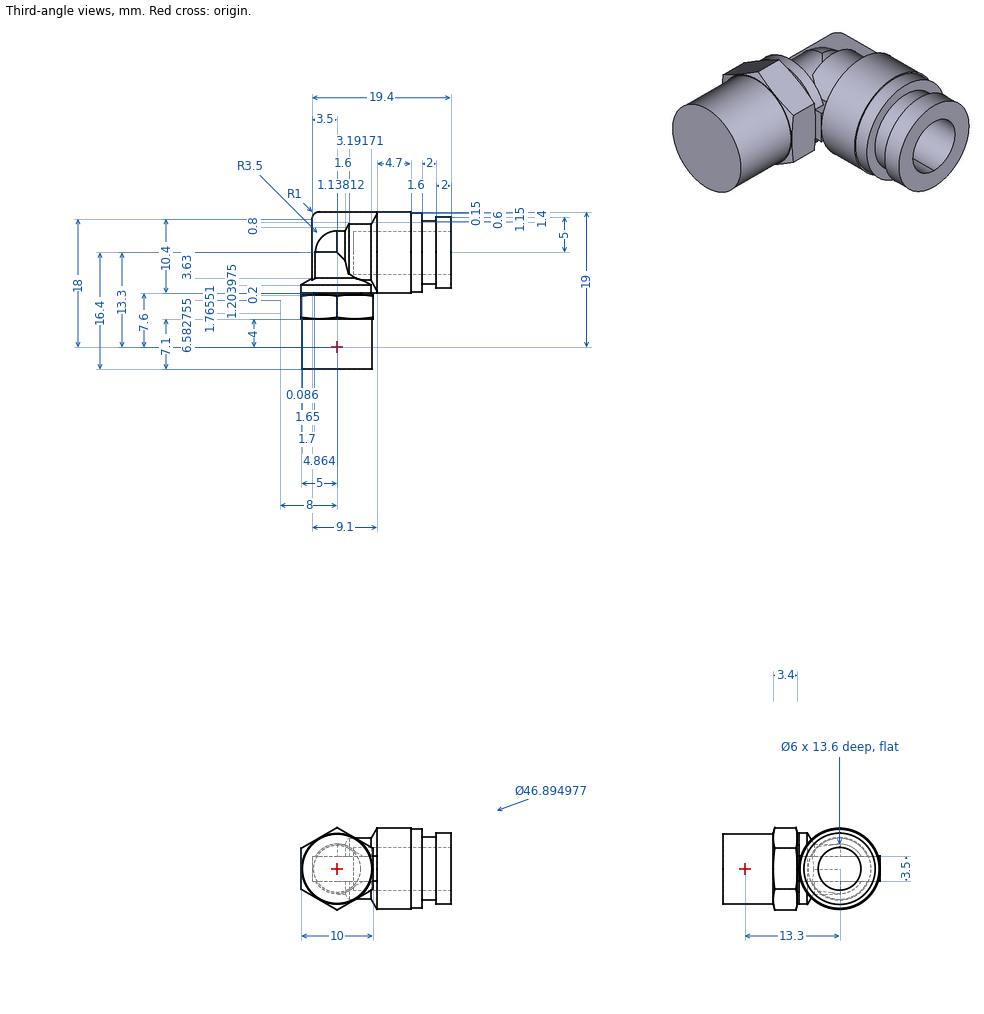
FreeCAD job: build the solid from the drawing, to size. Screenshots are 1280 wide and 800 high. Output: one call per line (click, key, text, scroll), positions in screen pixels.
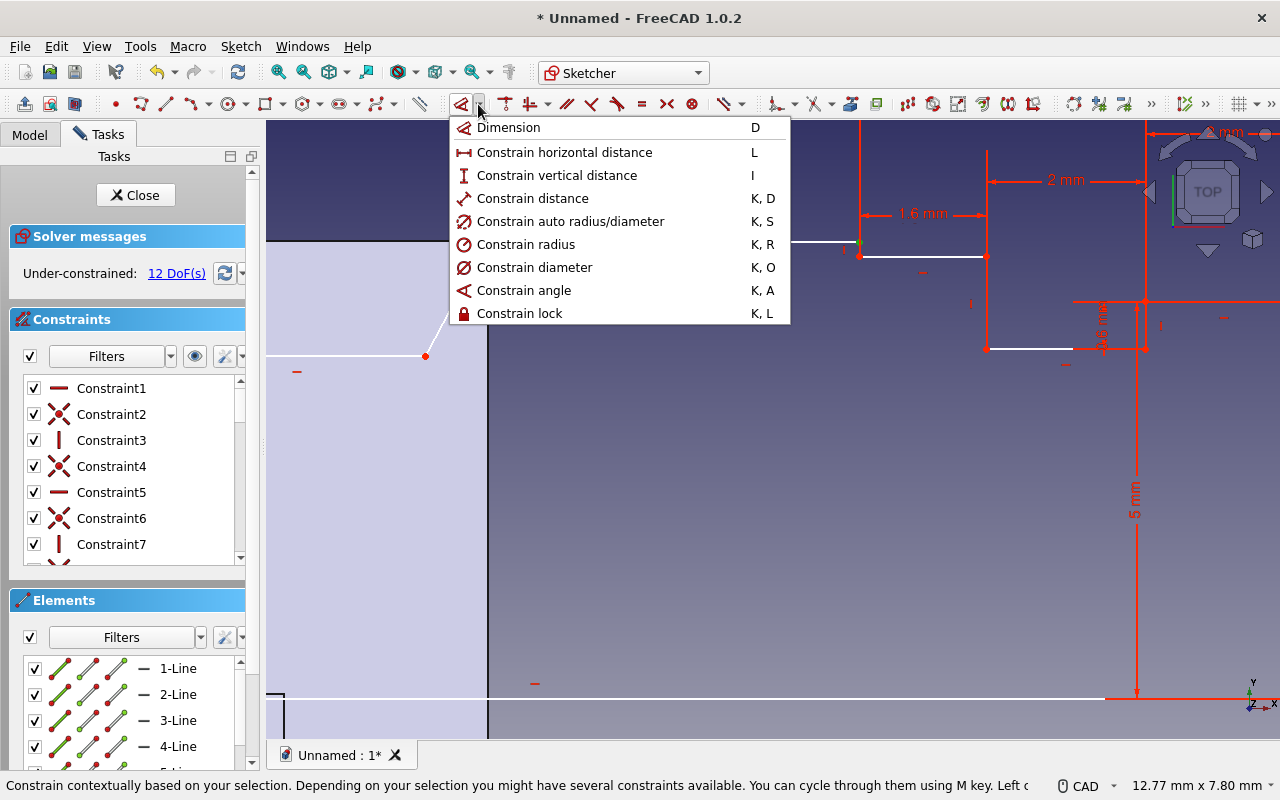
click(620, 176)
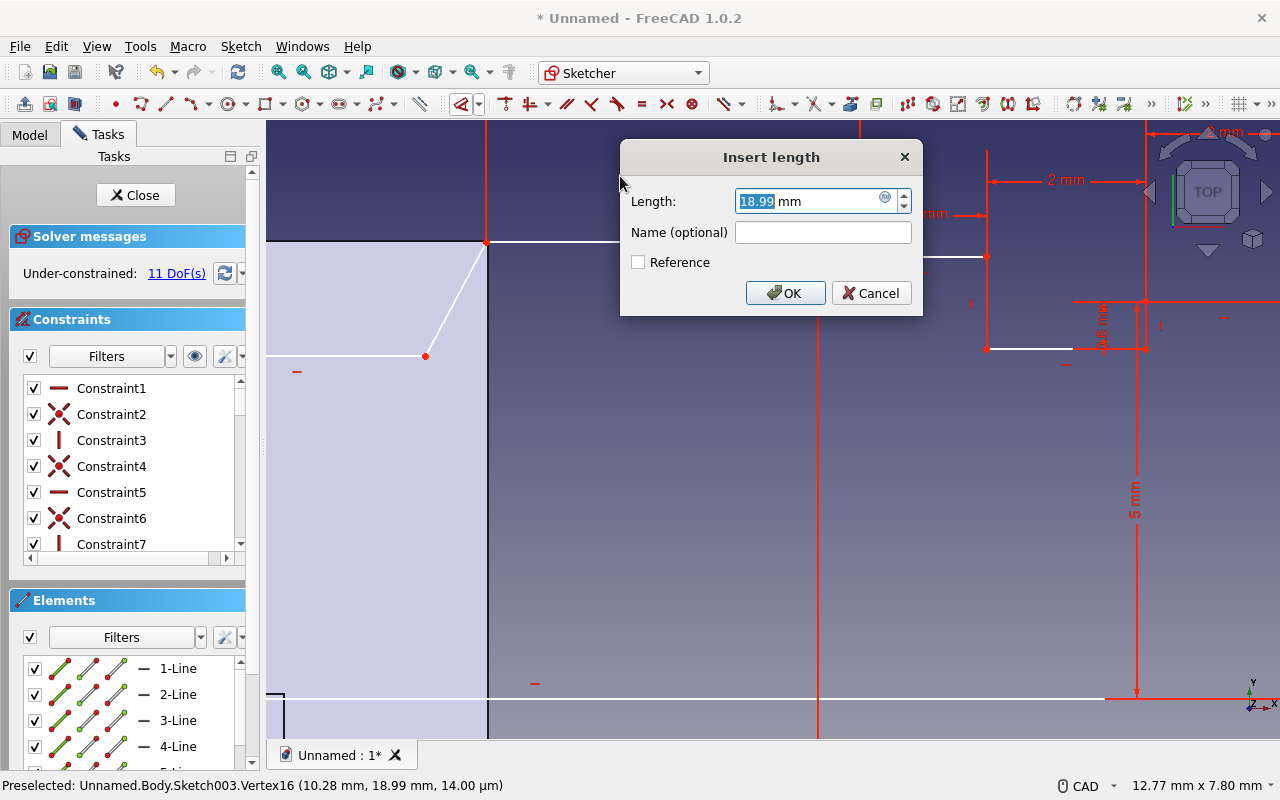
text(19)
key(Return)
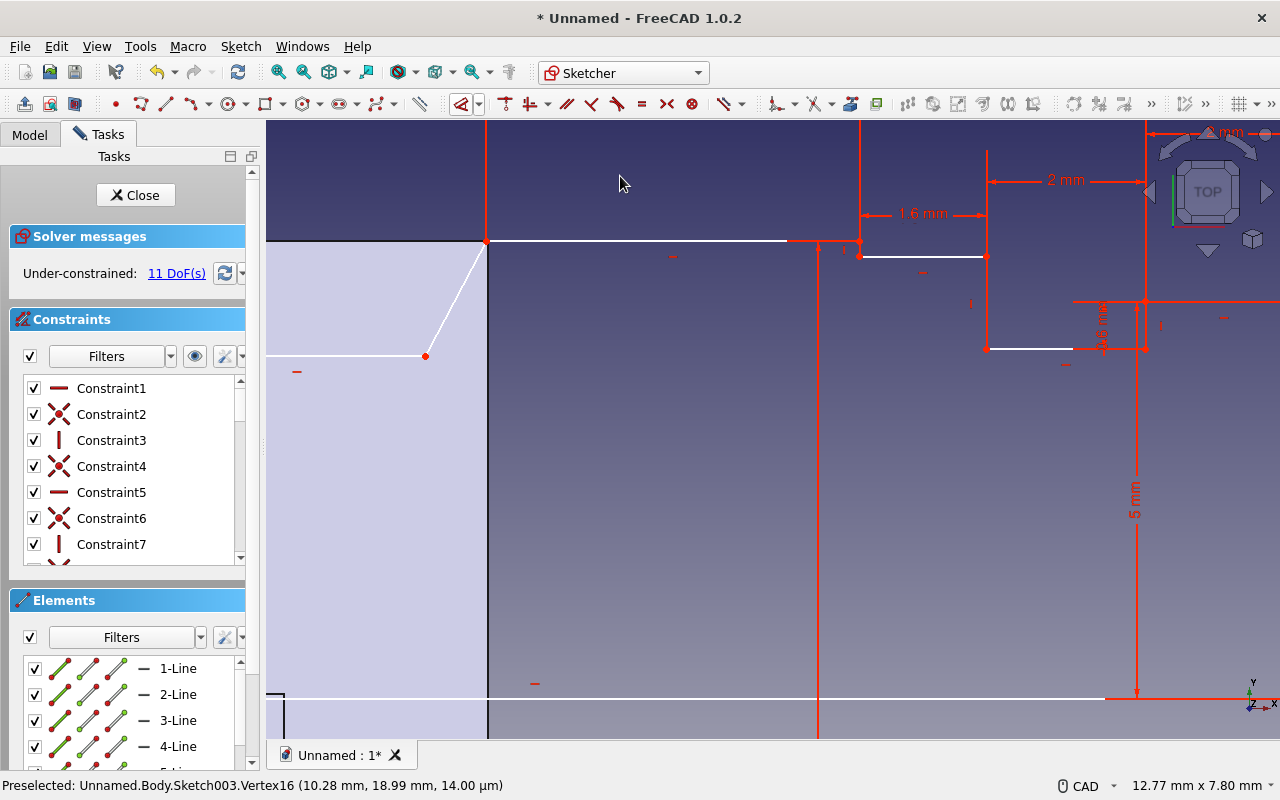
scroll(861, 244, down, 7)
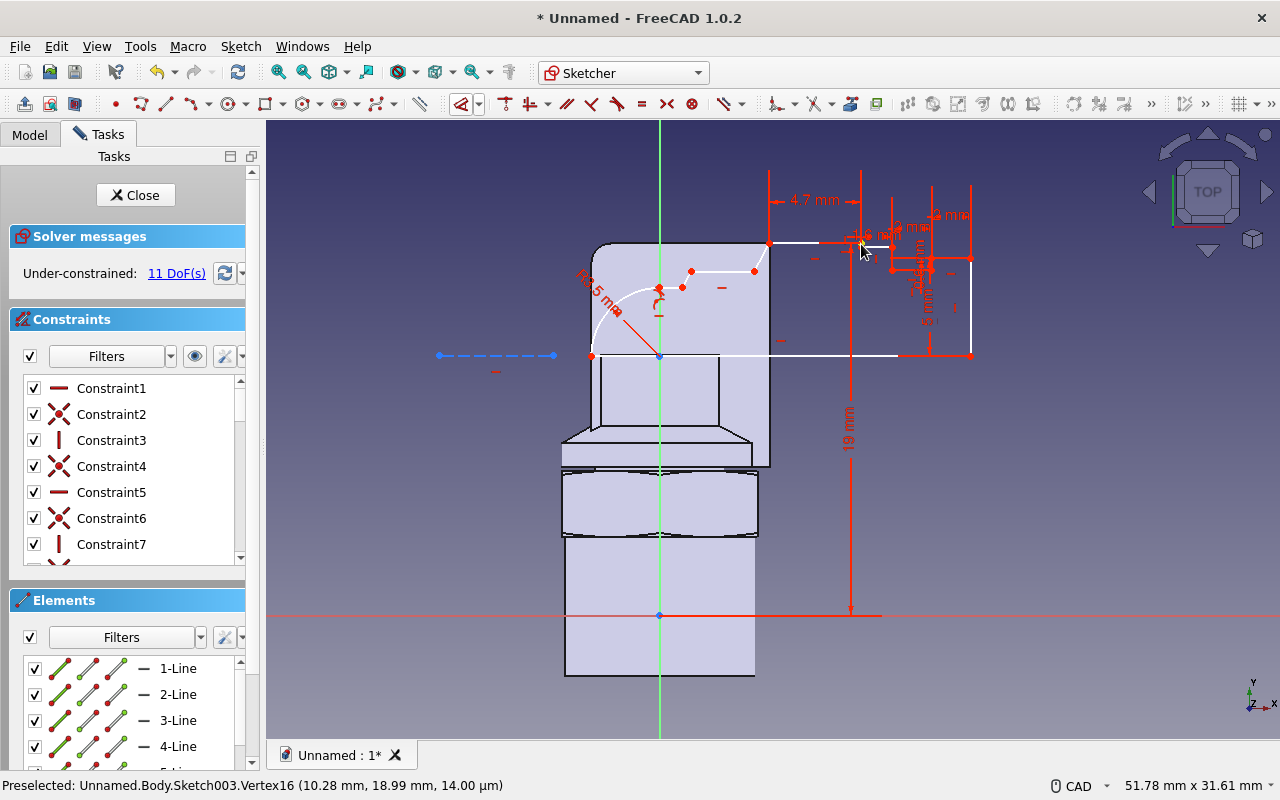
click(857, 356)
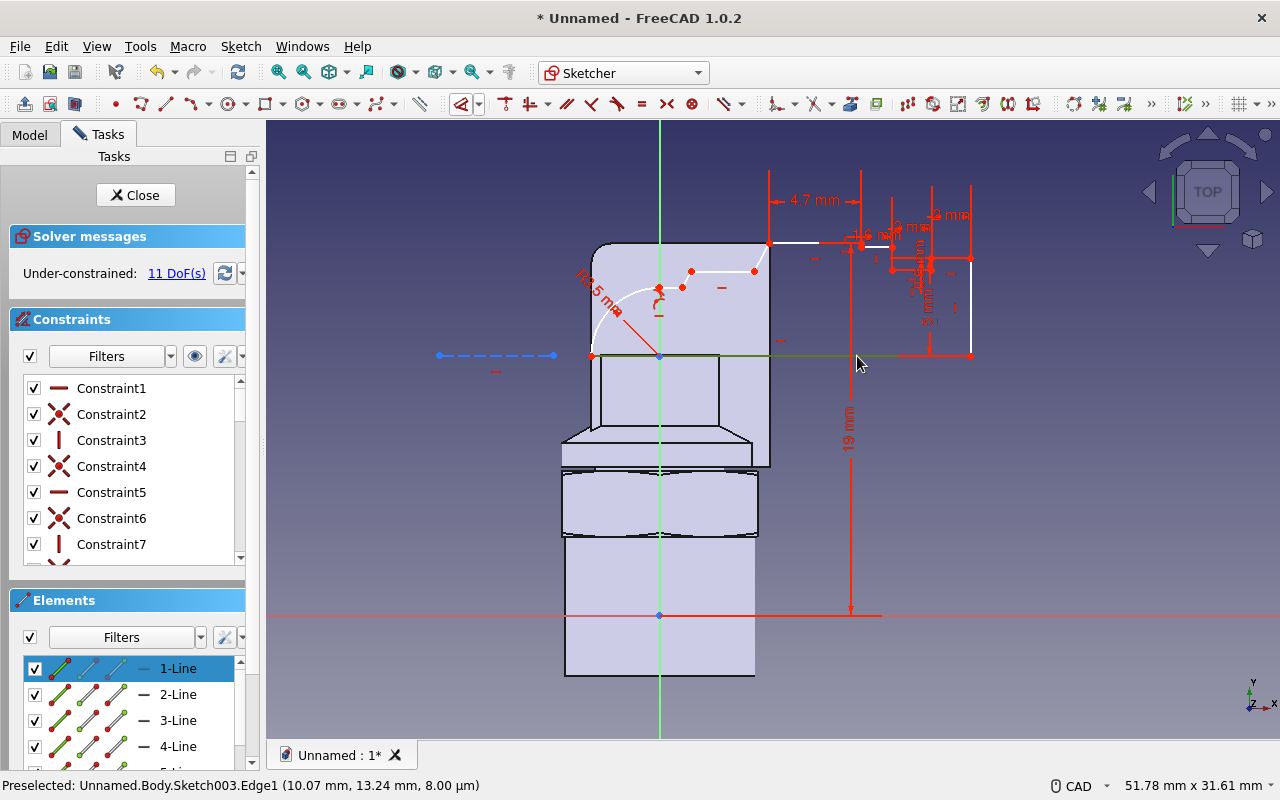
key(l)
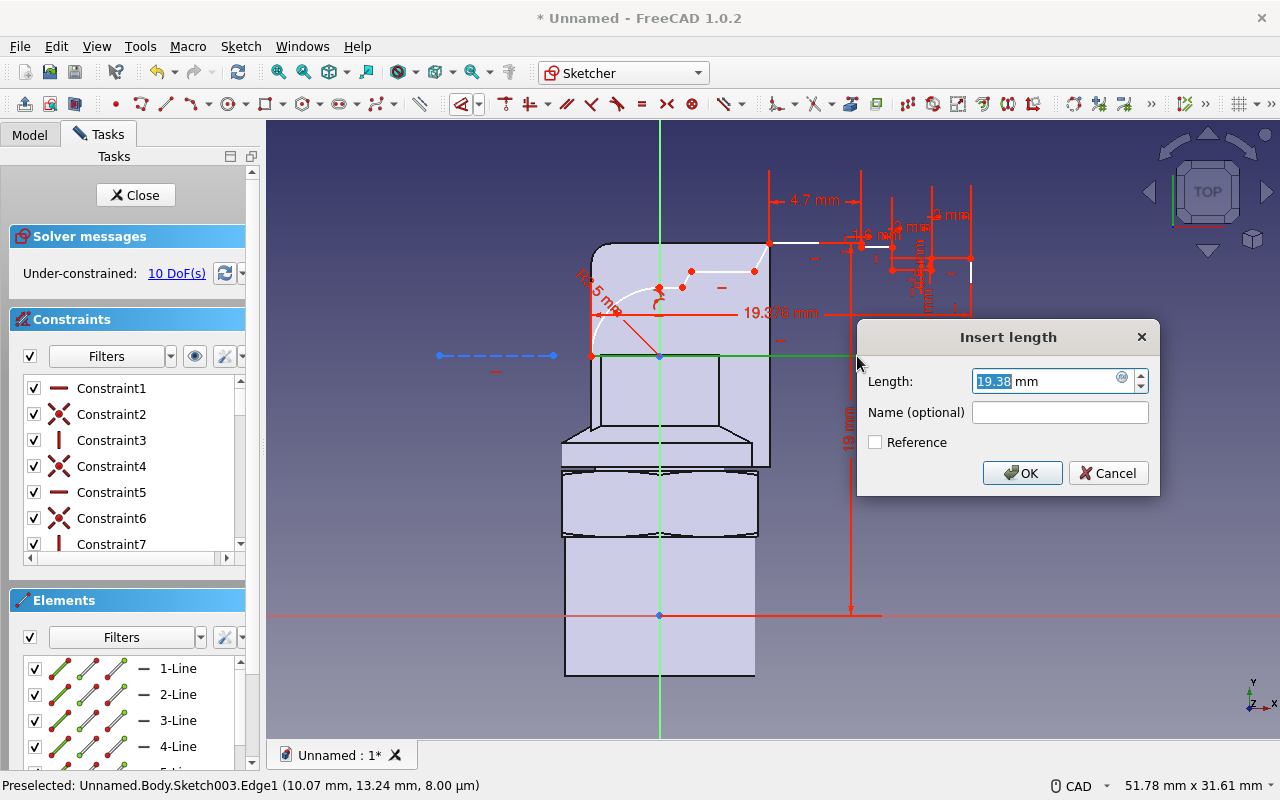
text(19.4)
key(Return)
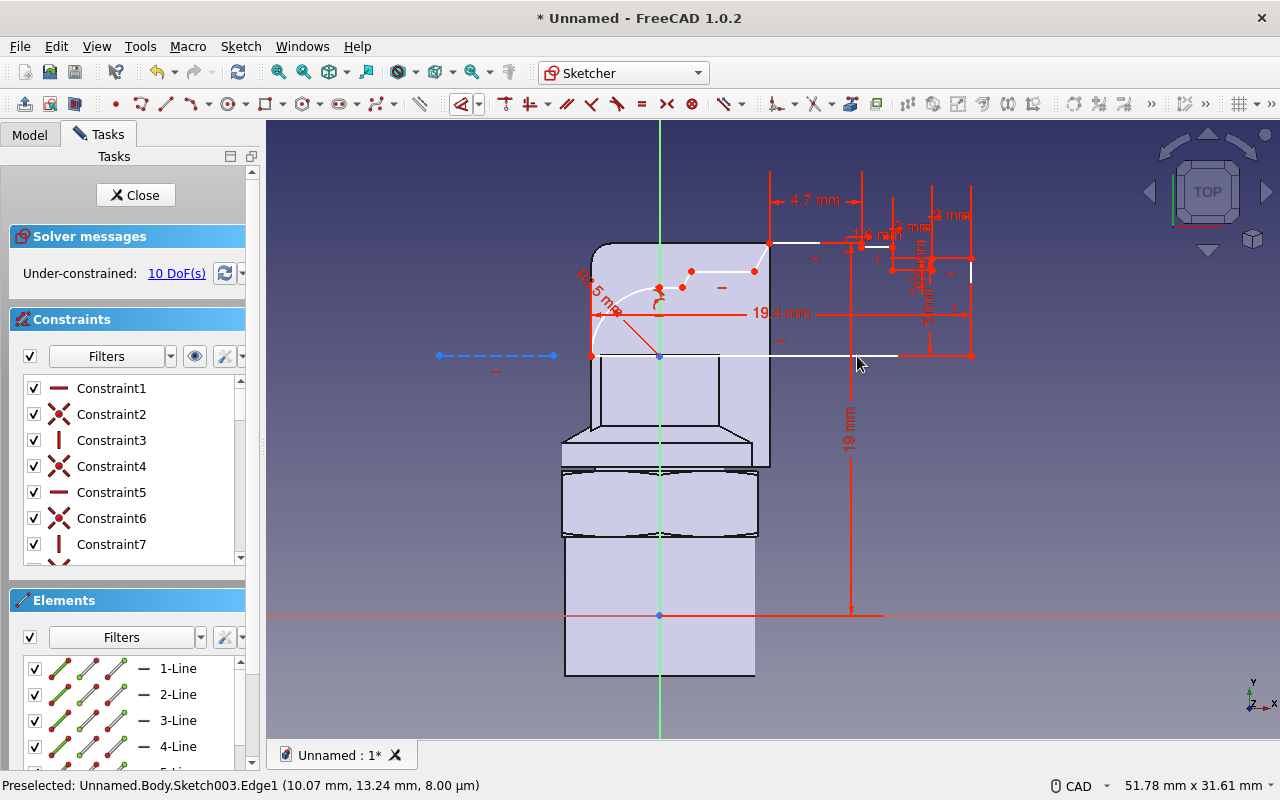
scroll(893, 261, up, 3)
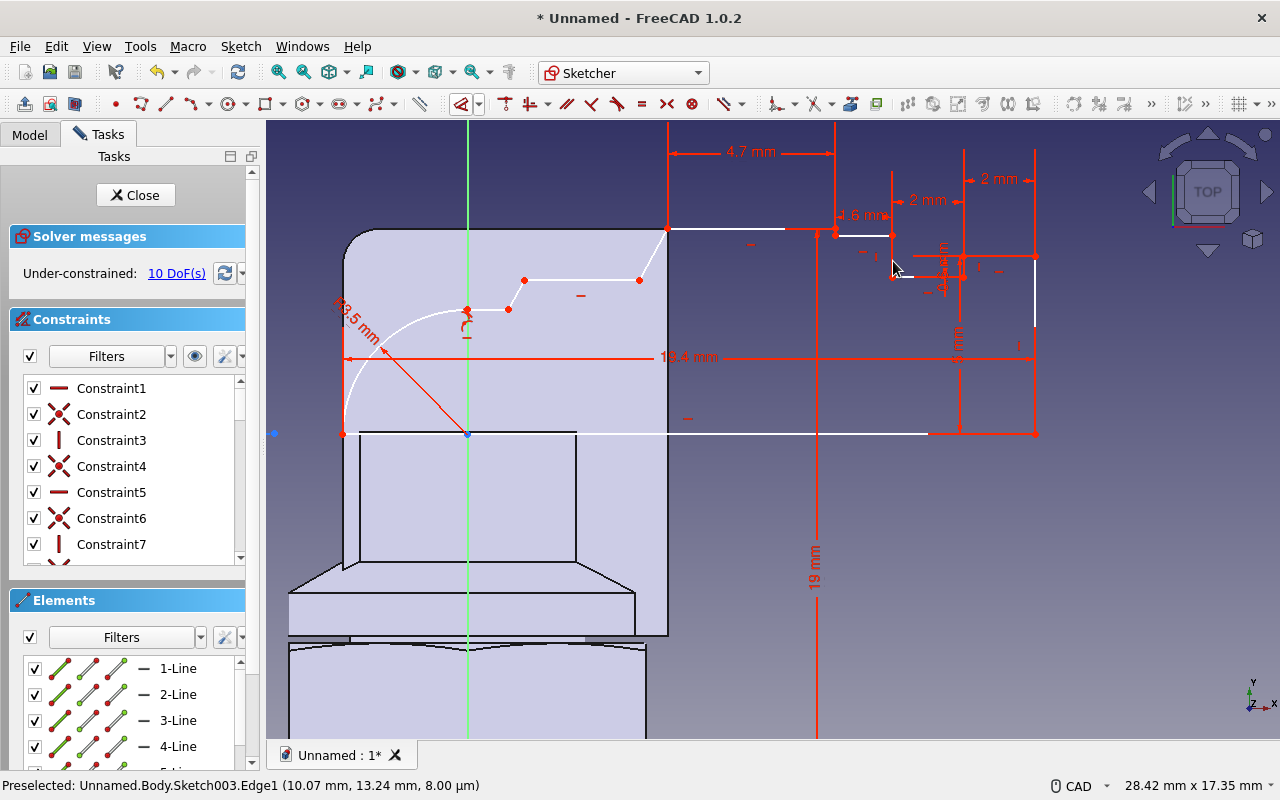
click(892, 261)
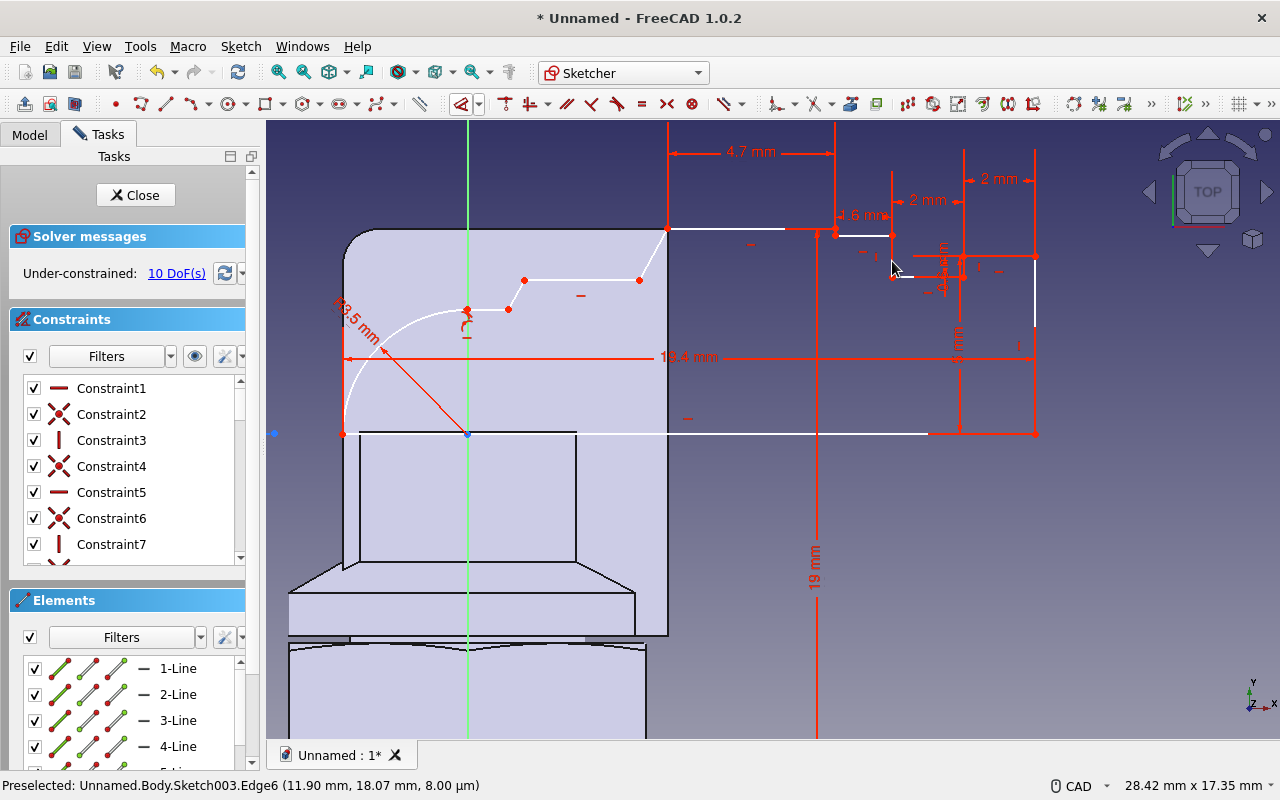
key(i)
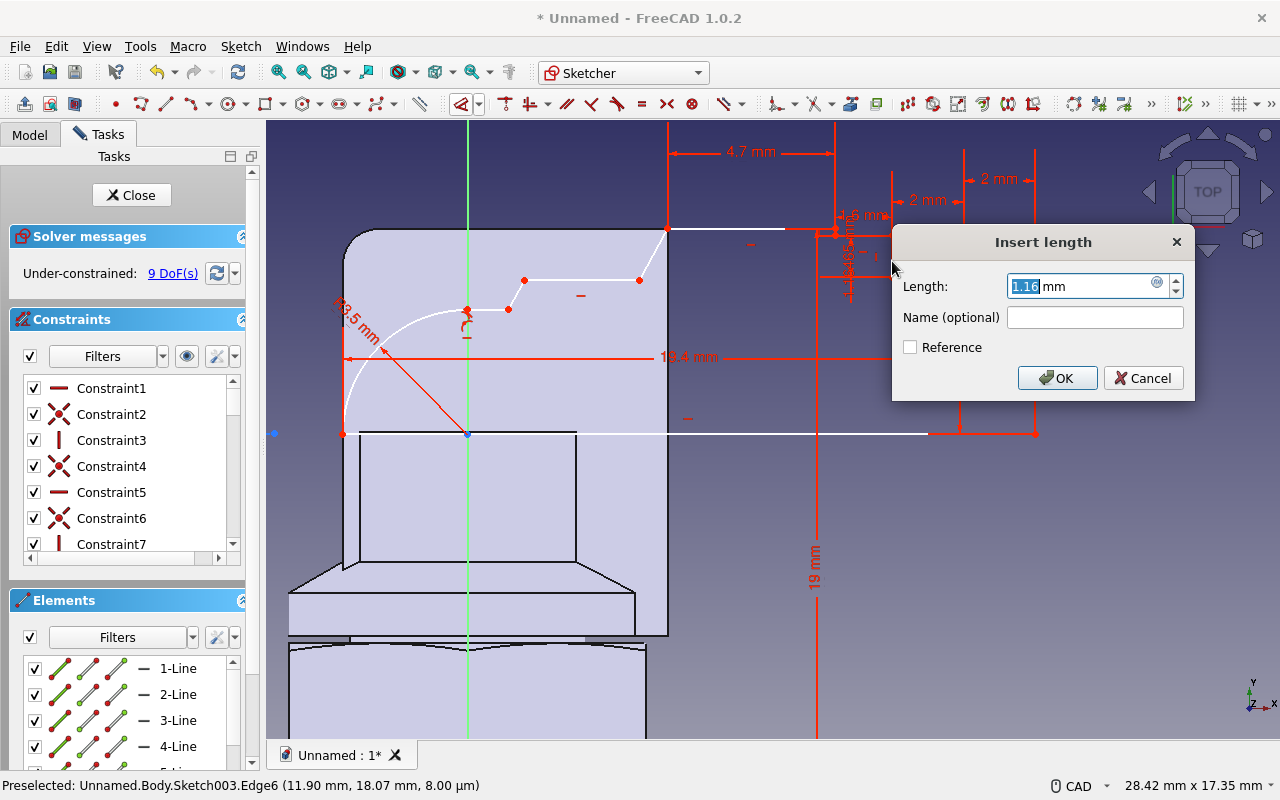
text(1.15)
key(Return)